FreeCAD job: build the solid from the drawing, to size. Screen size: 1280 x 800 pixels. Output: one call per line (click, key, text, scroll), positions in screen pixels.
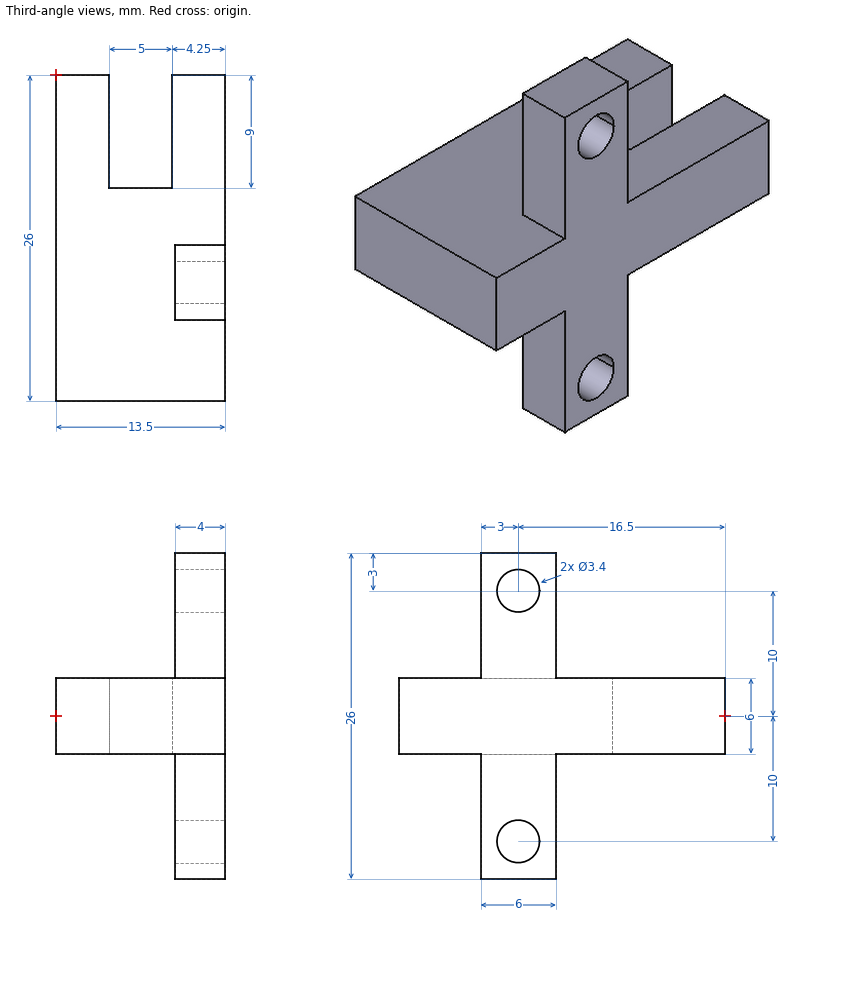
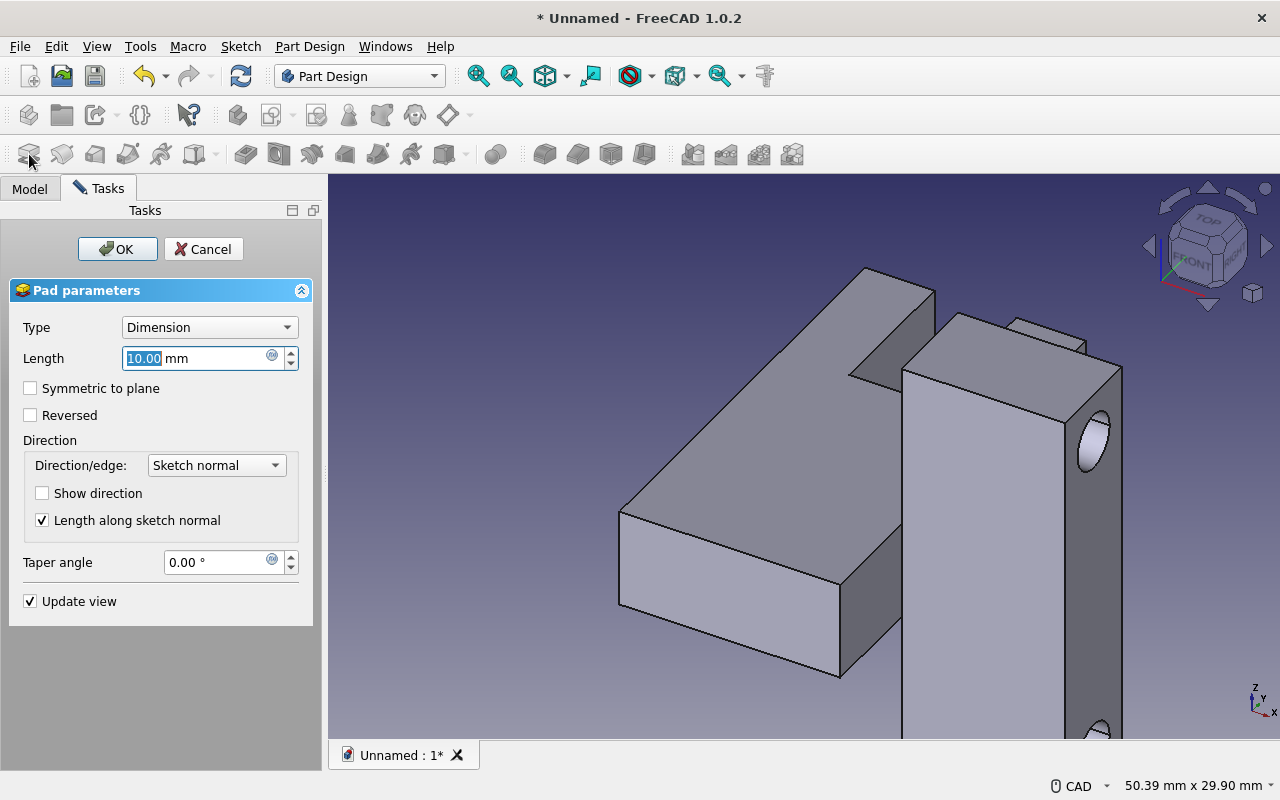
text(4)
key(Tab)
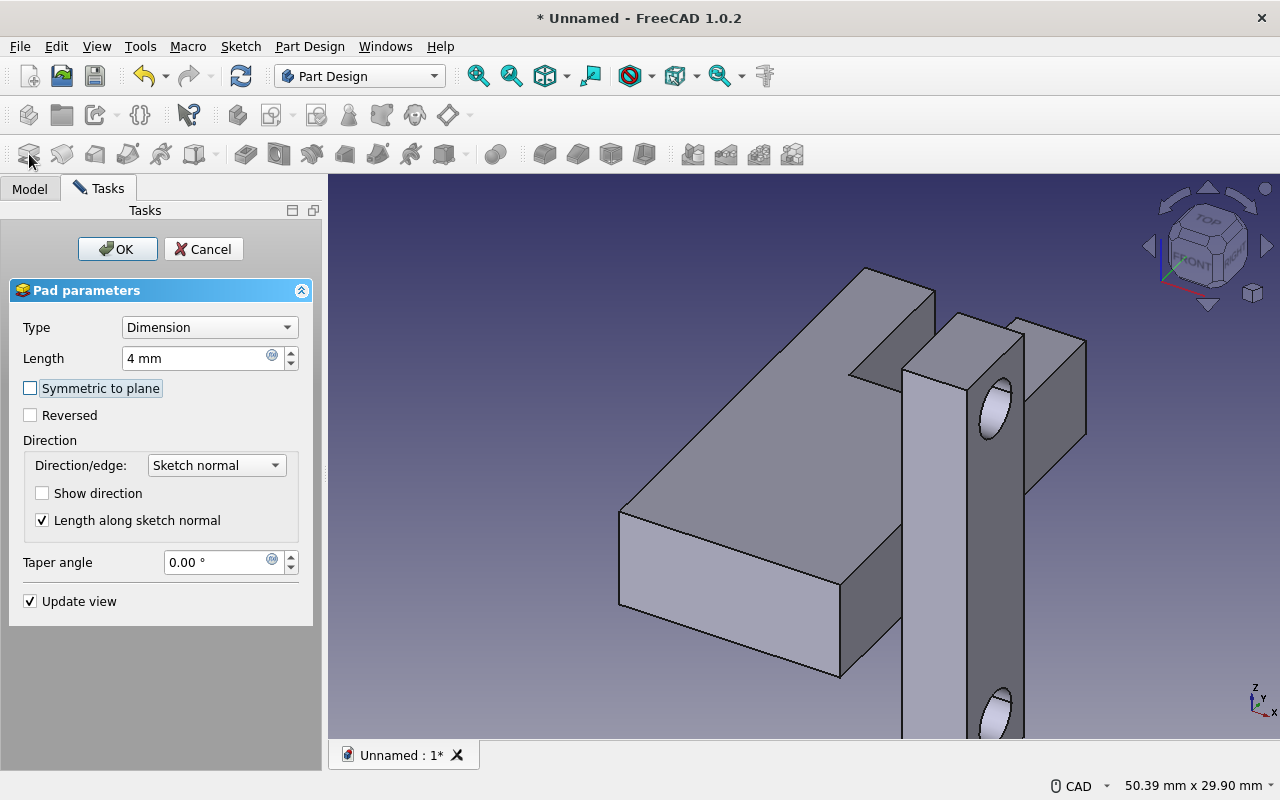
click(31, 415)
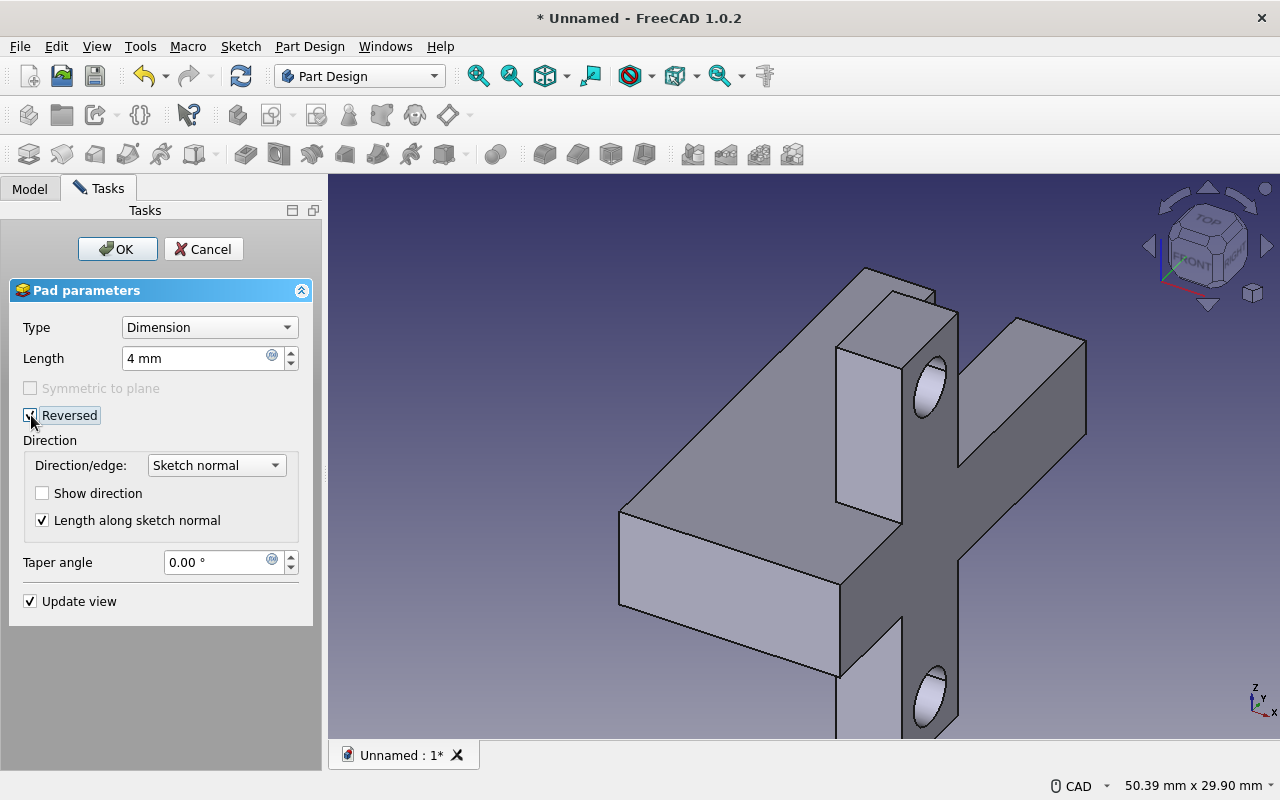
click(118, 249)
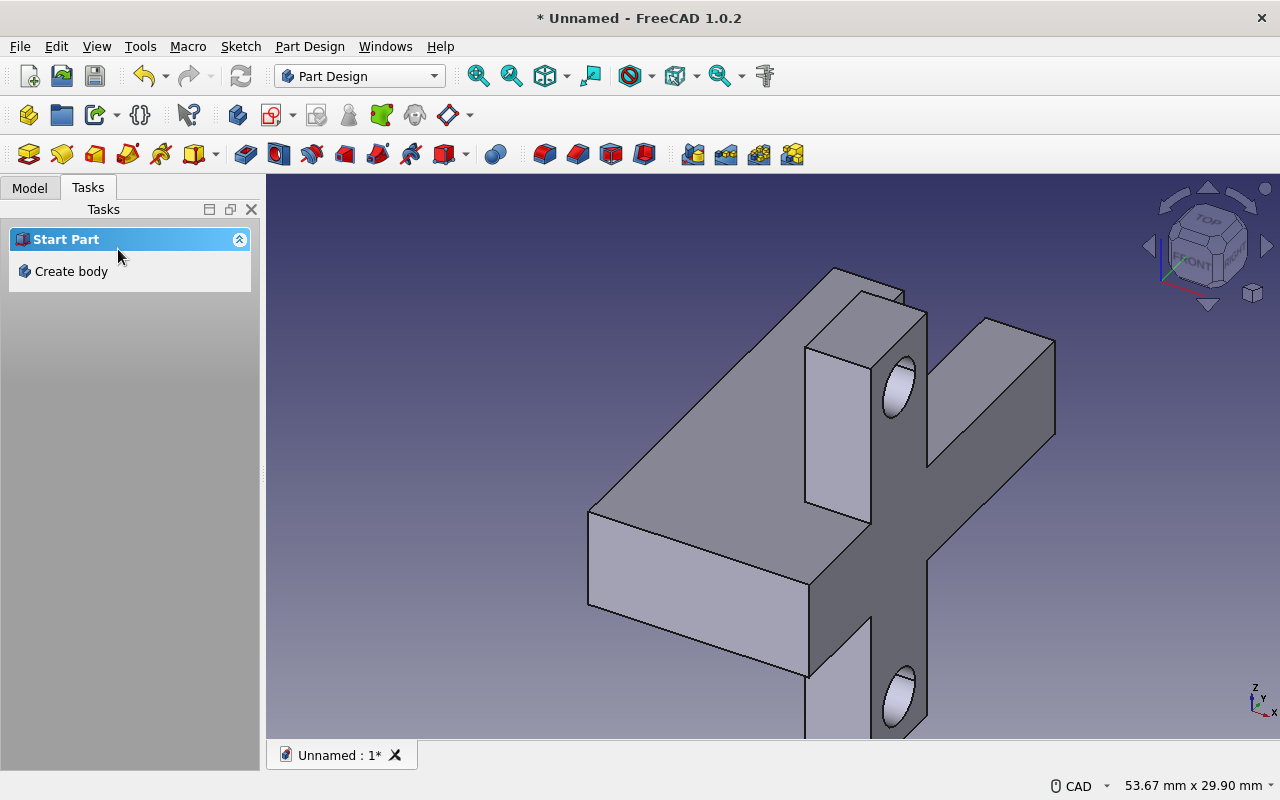
key(0)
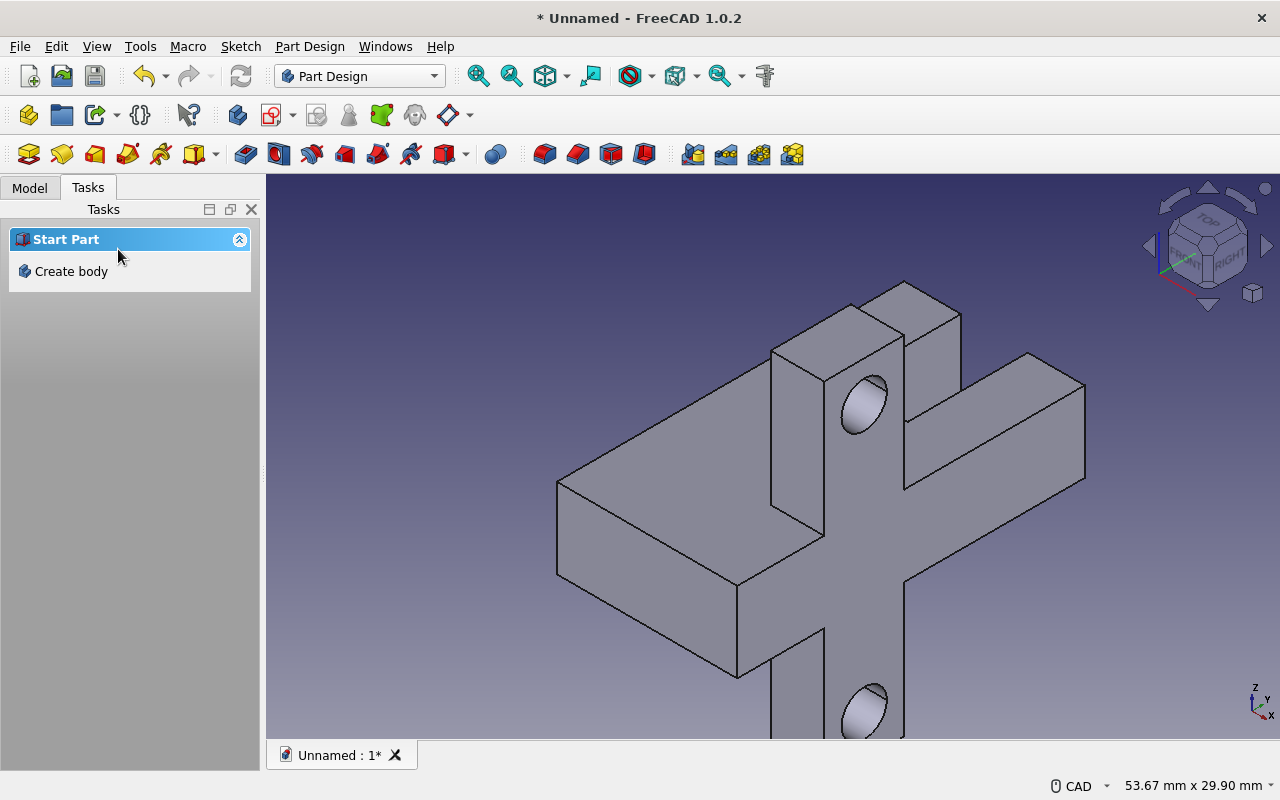
click(479, 76)